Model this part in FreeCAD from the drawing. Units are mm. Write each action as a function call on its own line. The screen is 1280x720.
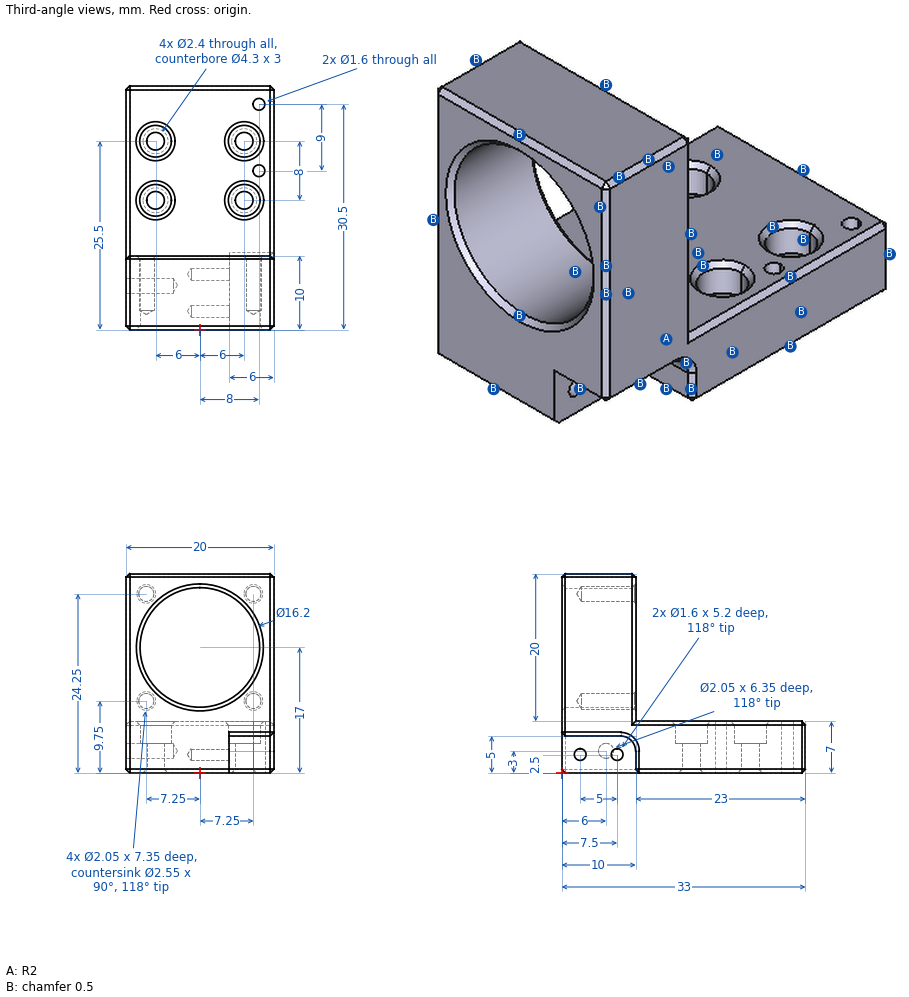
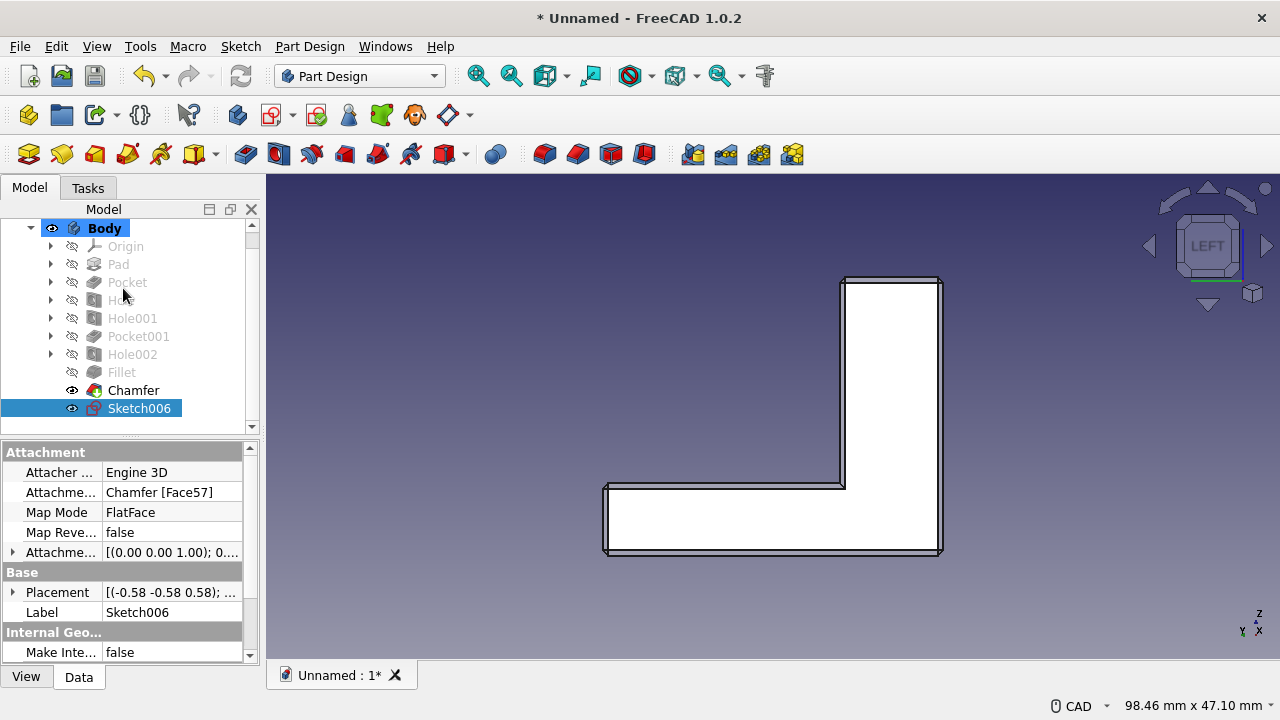
click(279, 154)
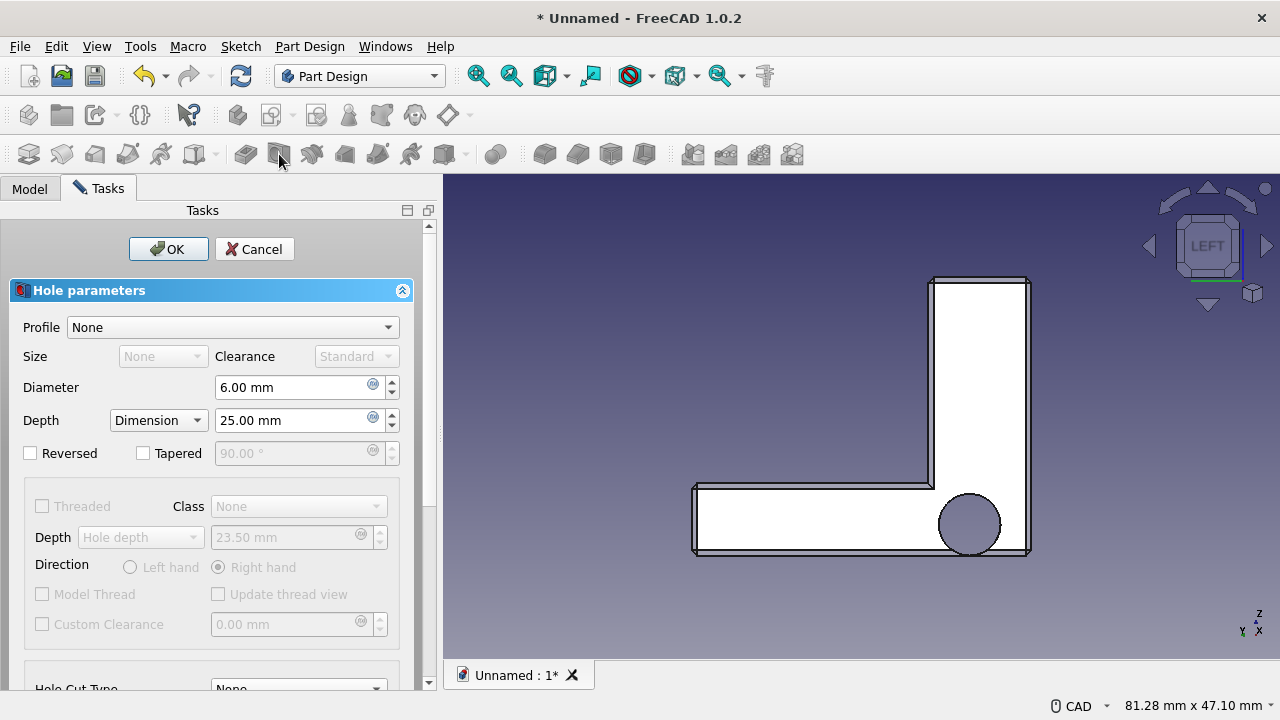
triple_click(300, 388)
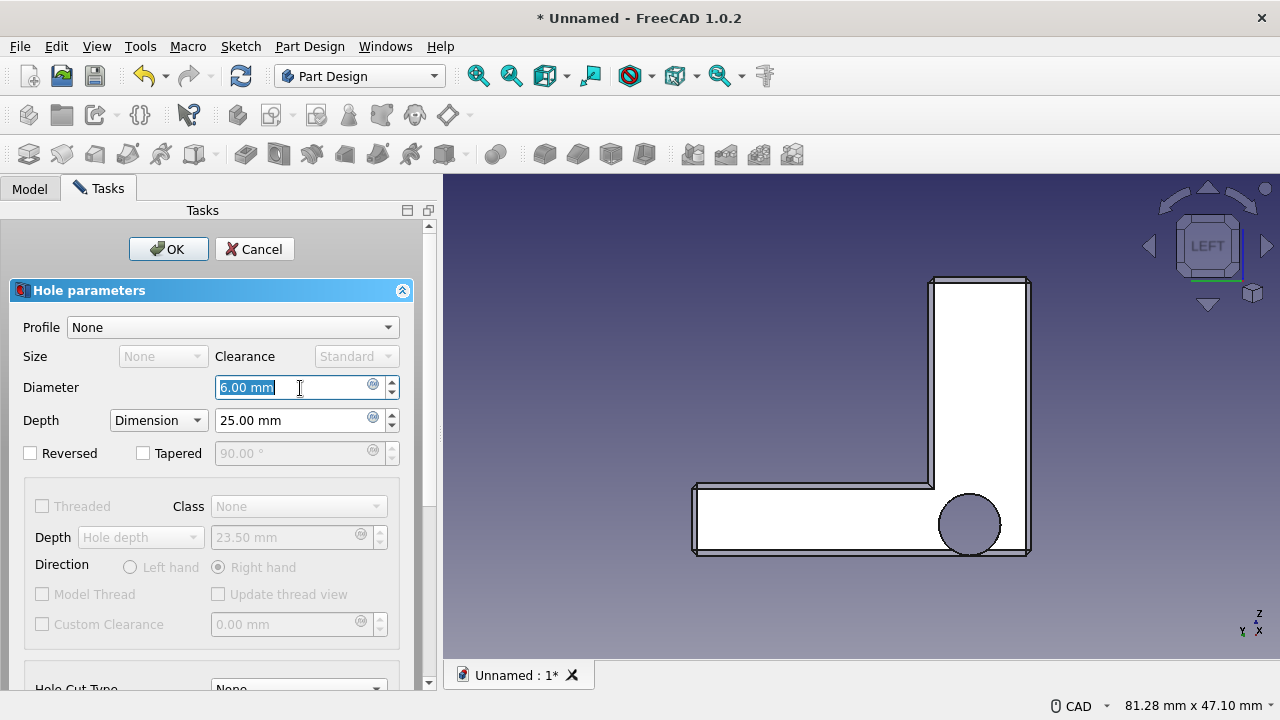
text(2.05)
key(Tab)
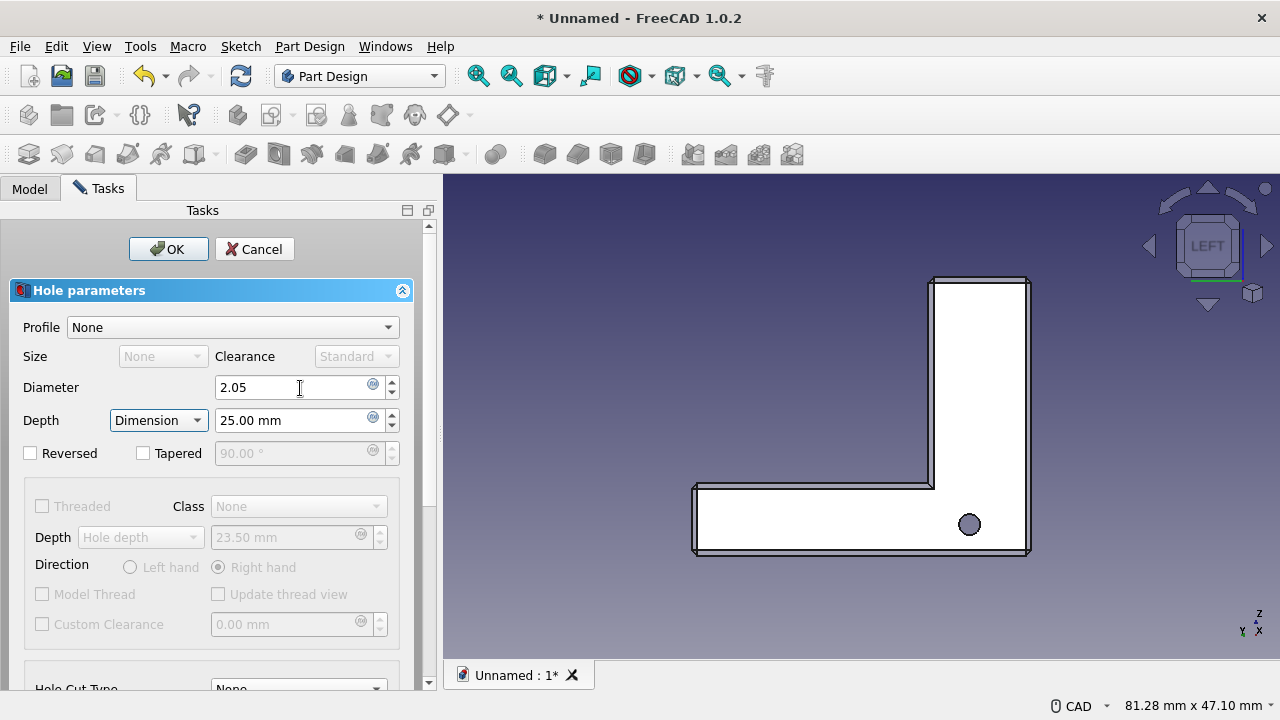
triple_click(300, 420)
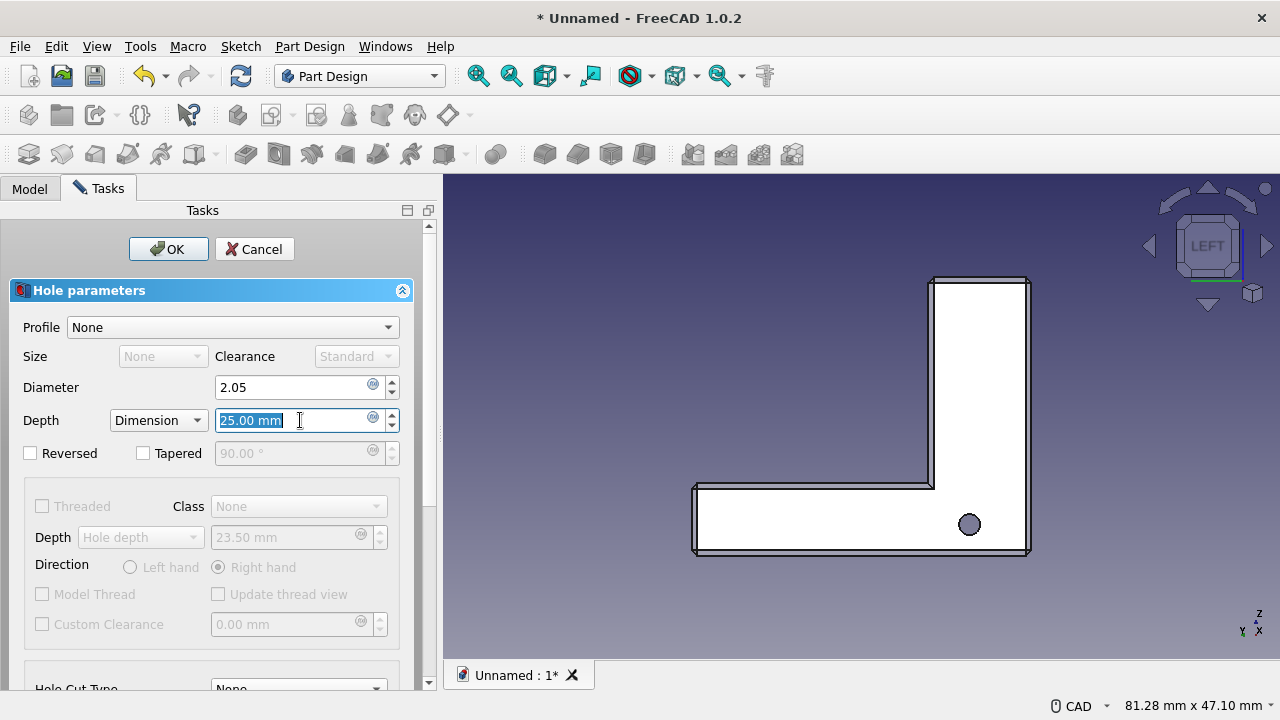
text(6.35)
key(Tab)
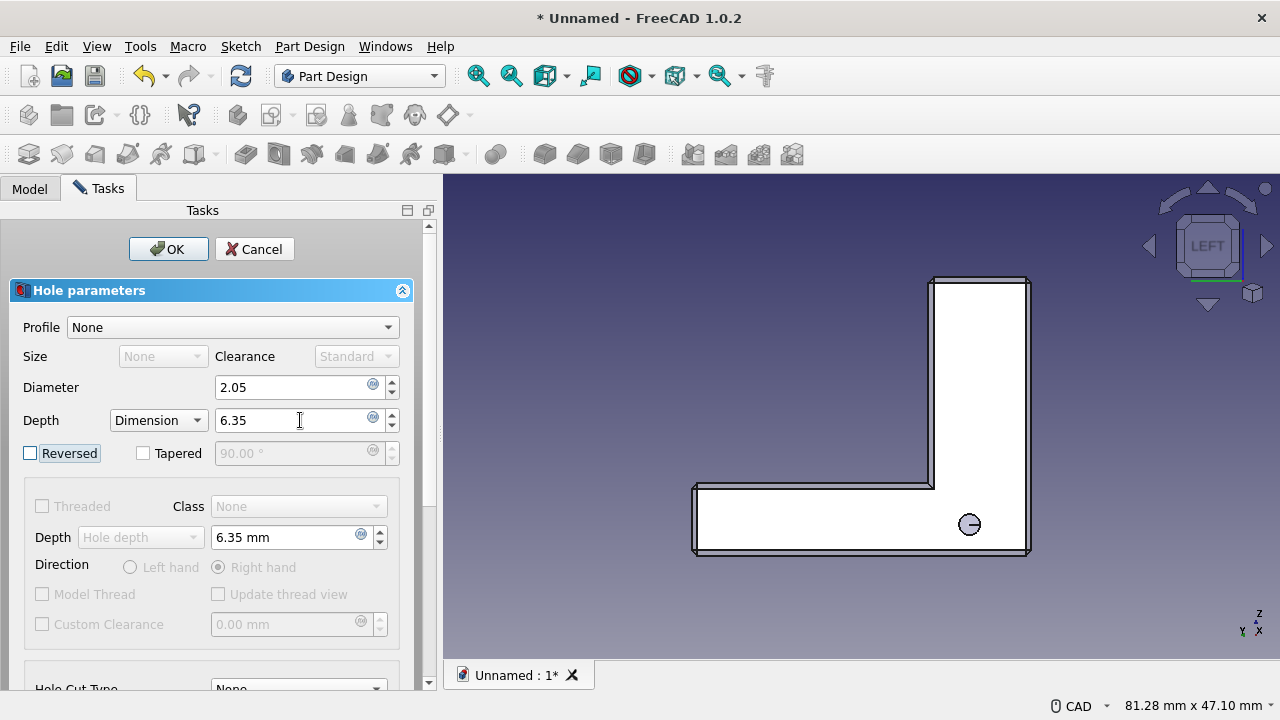
click(169, 249)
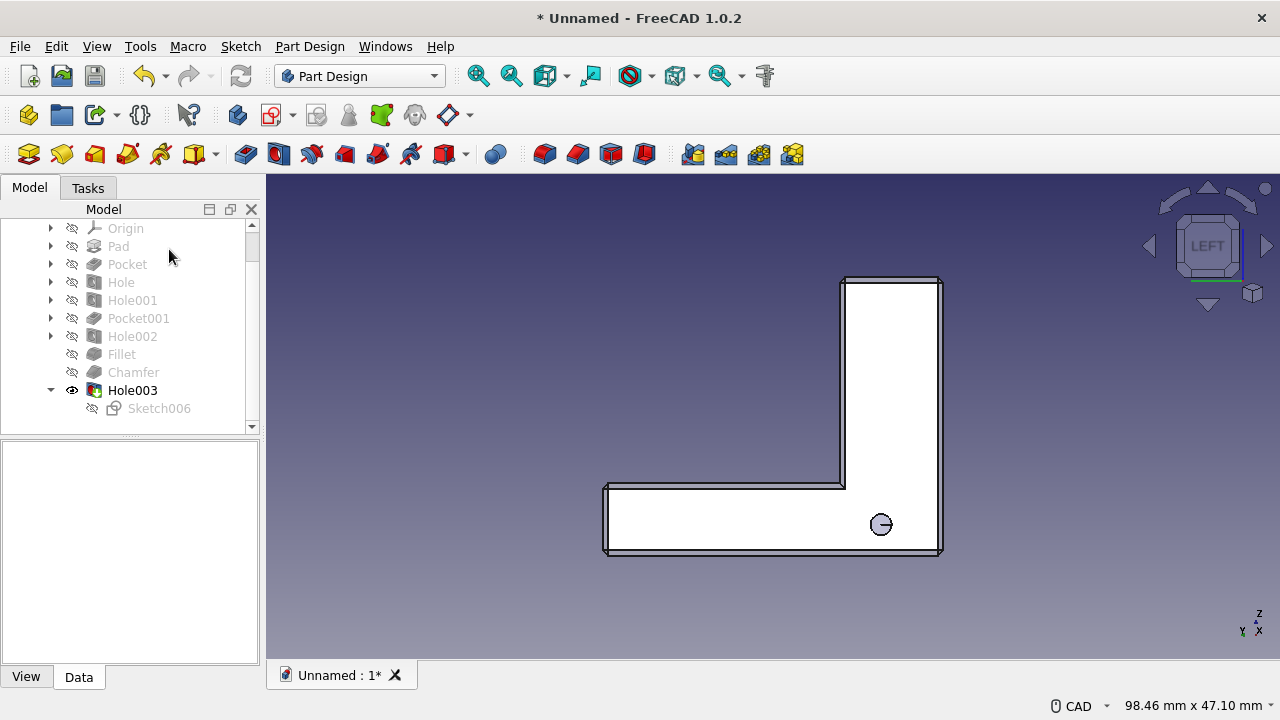
key(0)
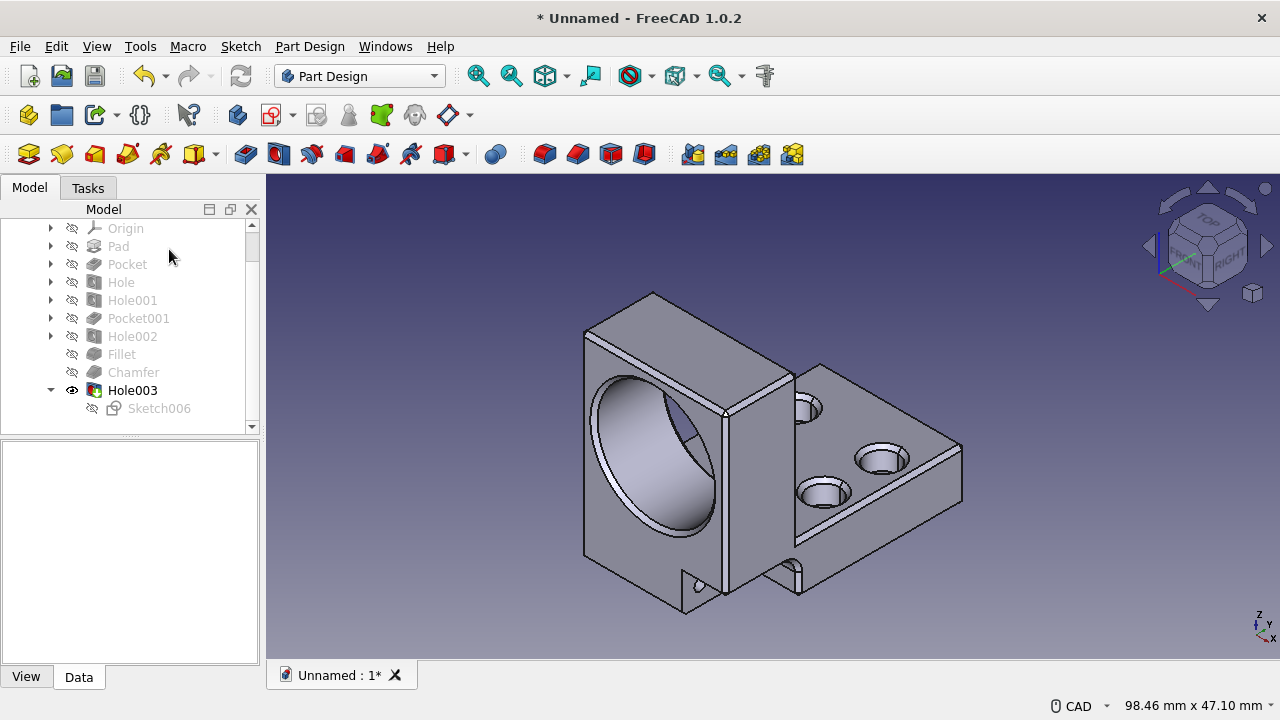
click(808, 450)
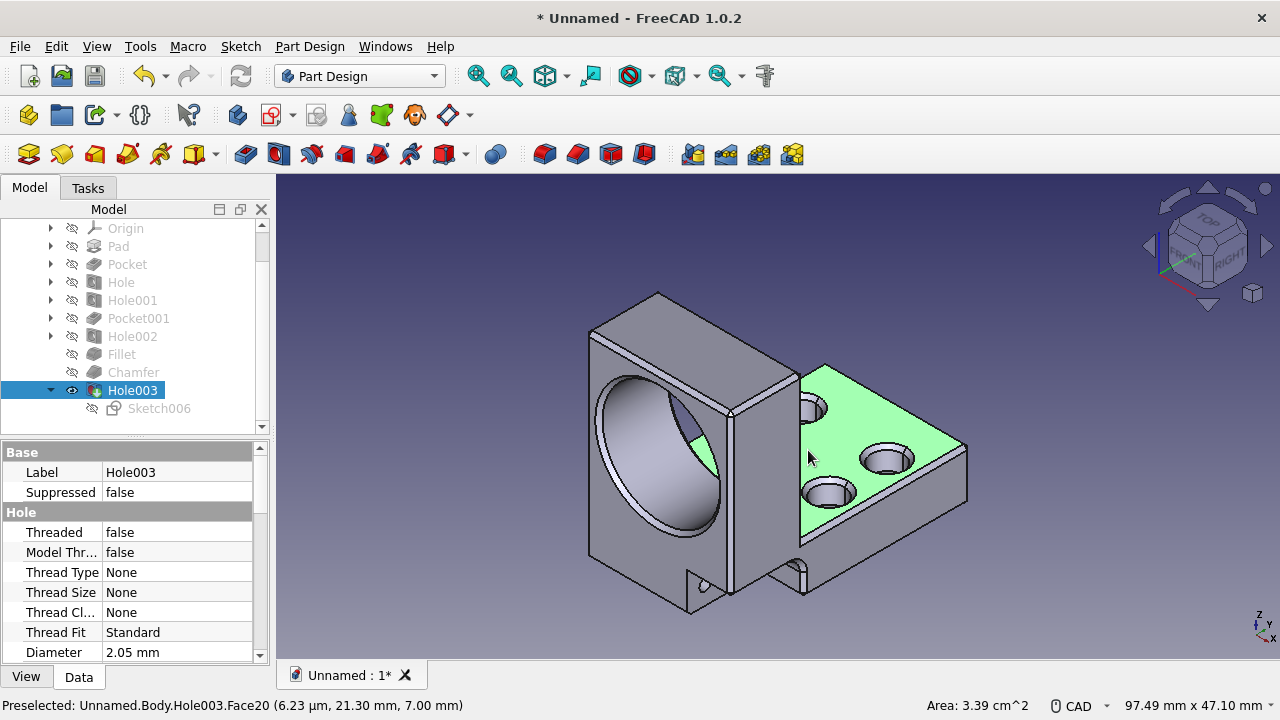
click(270, 116)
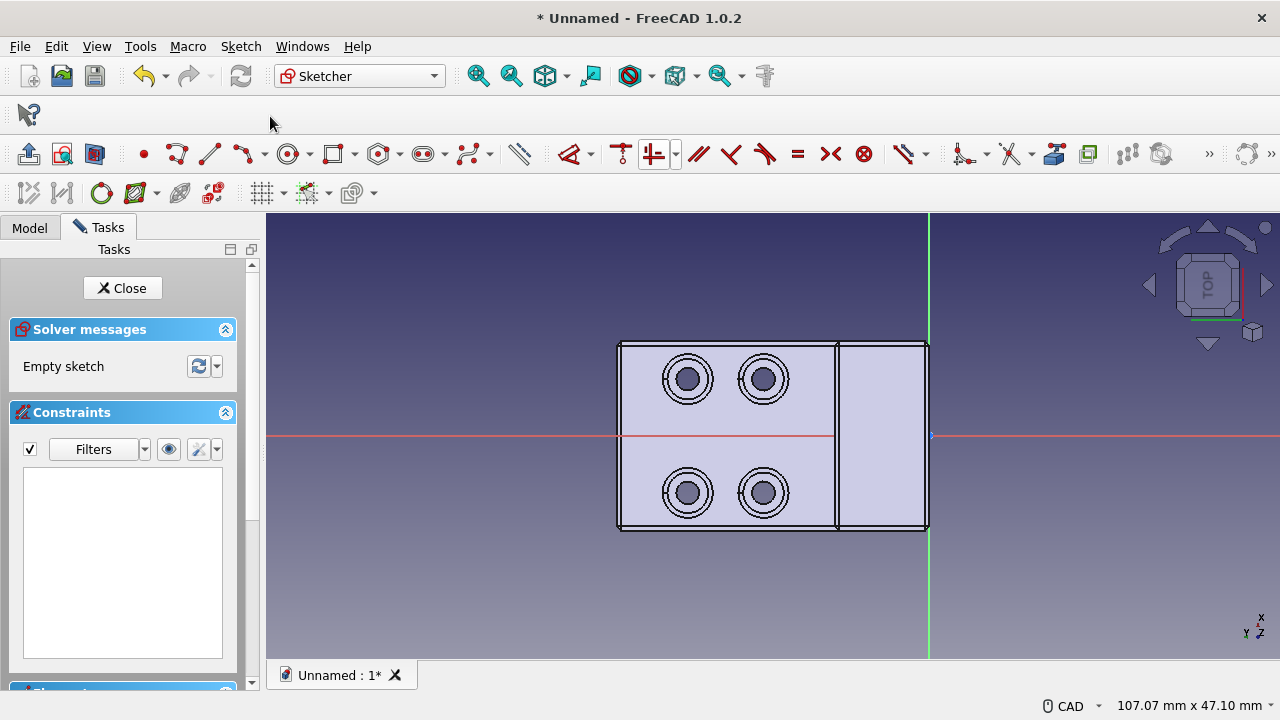
scroll(679, 345, up, 9)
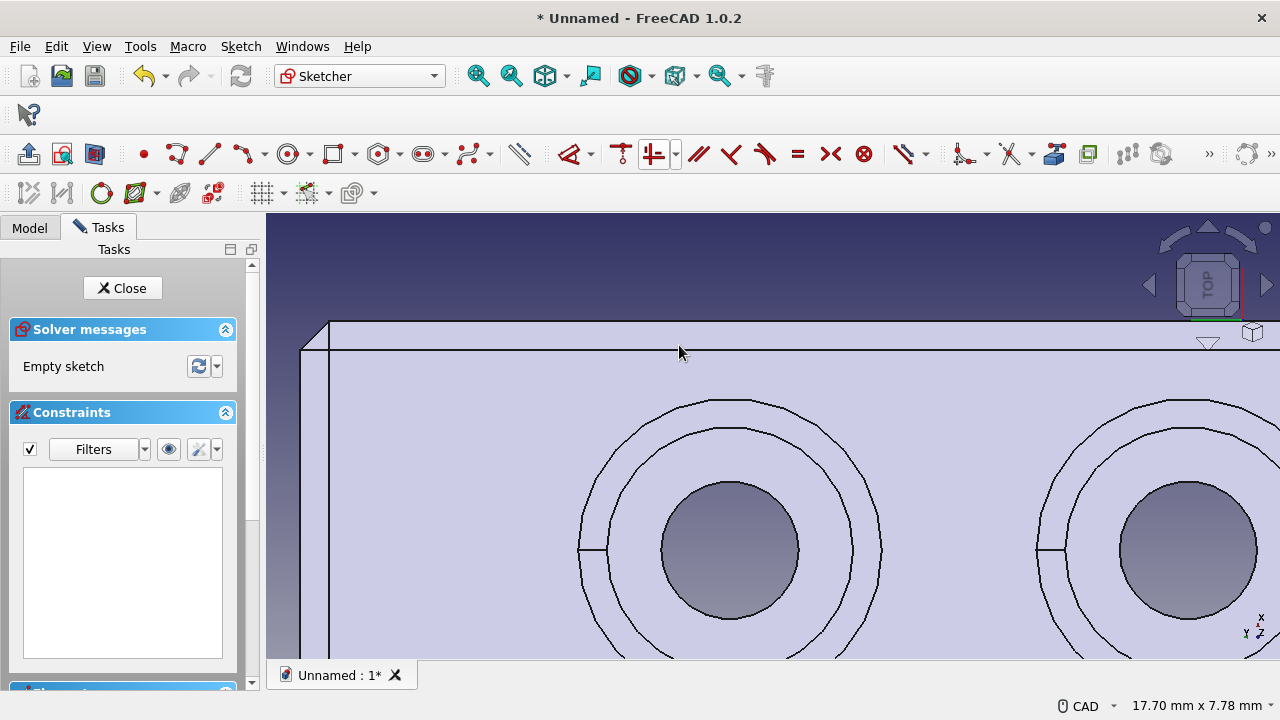
key(g)
key(c)